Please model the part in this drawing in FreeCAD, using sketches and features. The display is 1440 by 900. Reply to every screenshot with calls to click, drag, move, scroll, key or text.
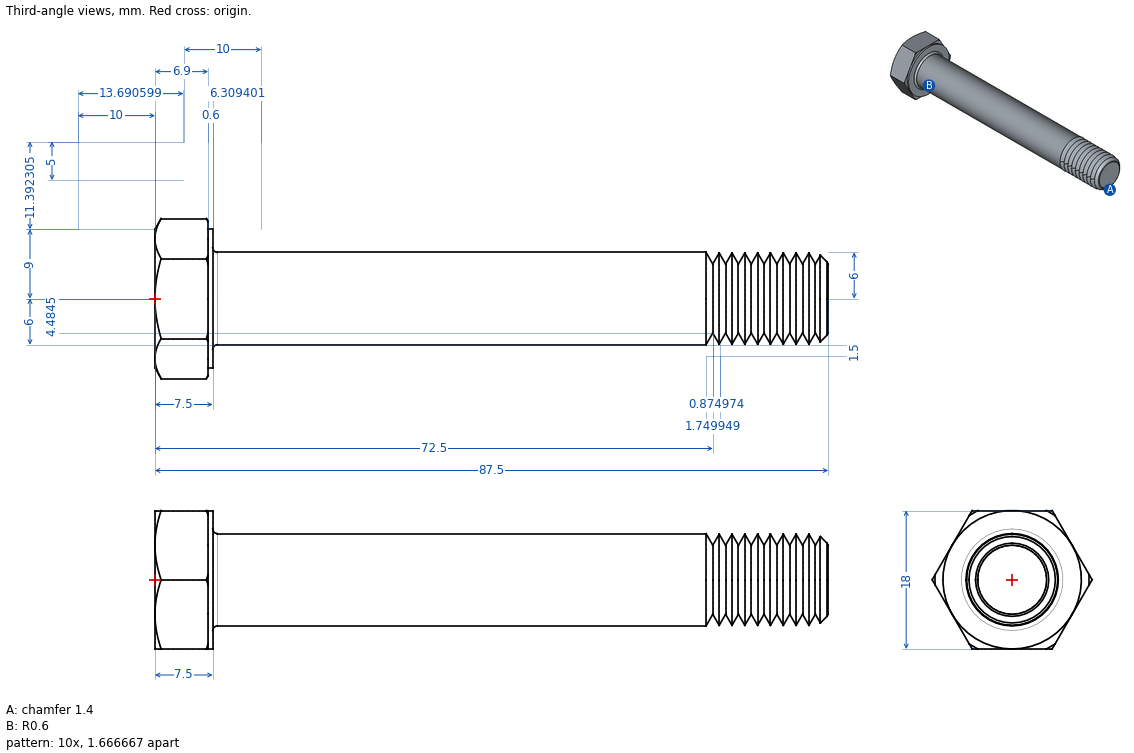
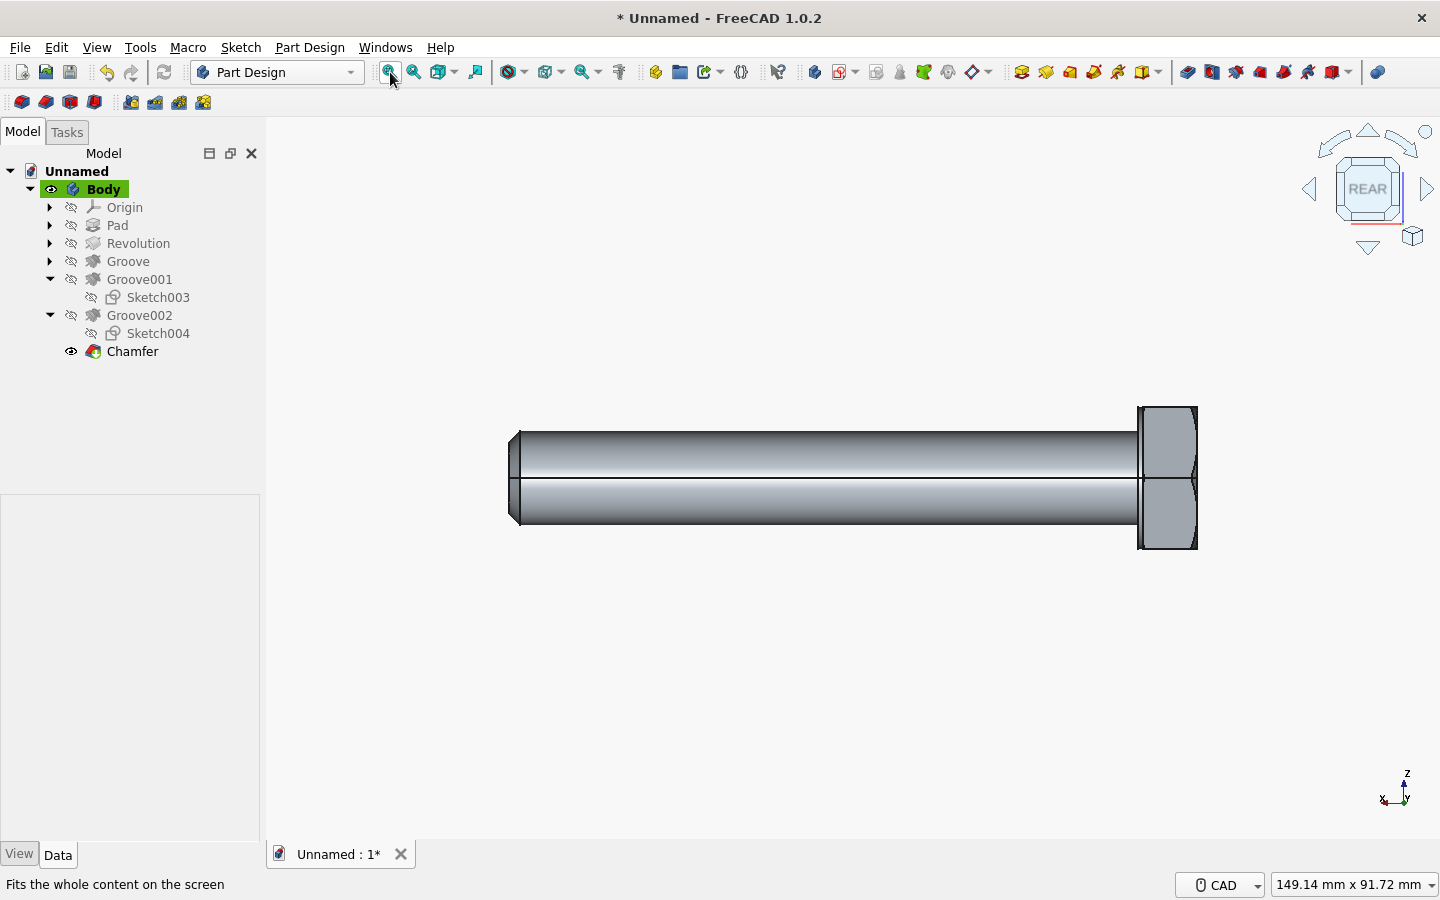
key(6)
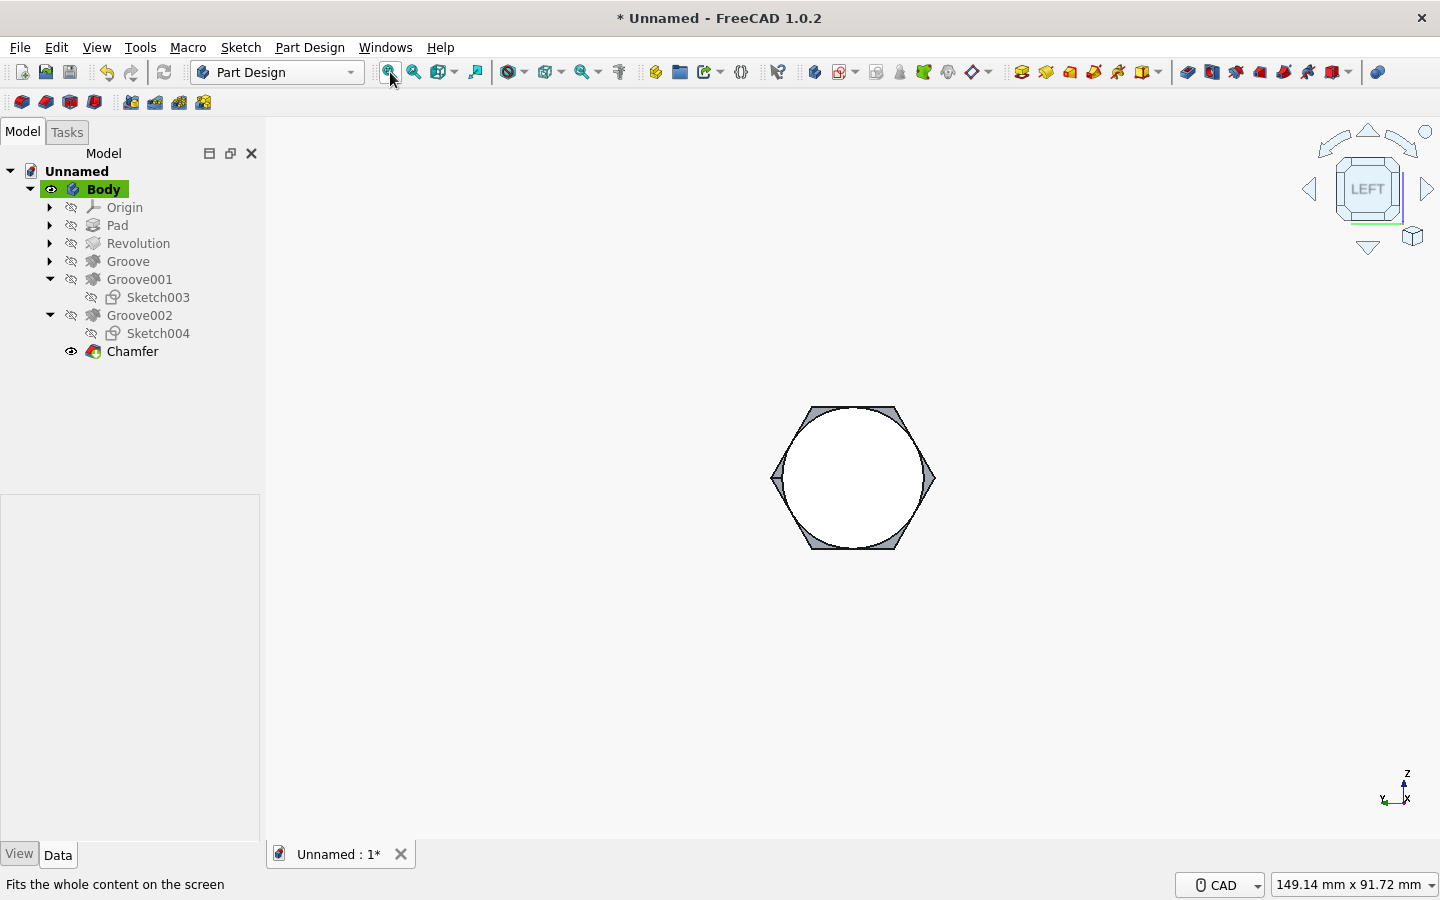
click(390, 72)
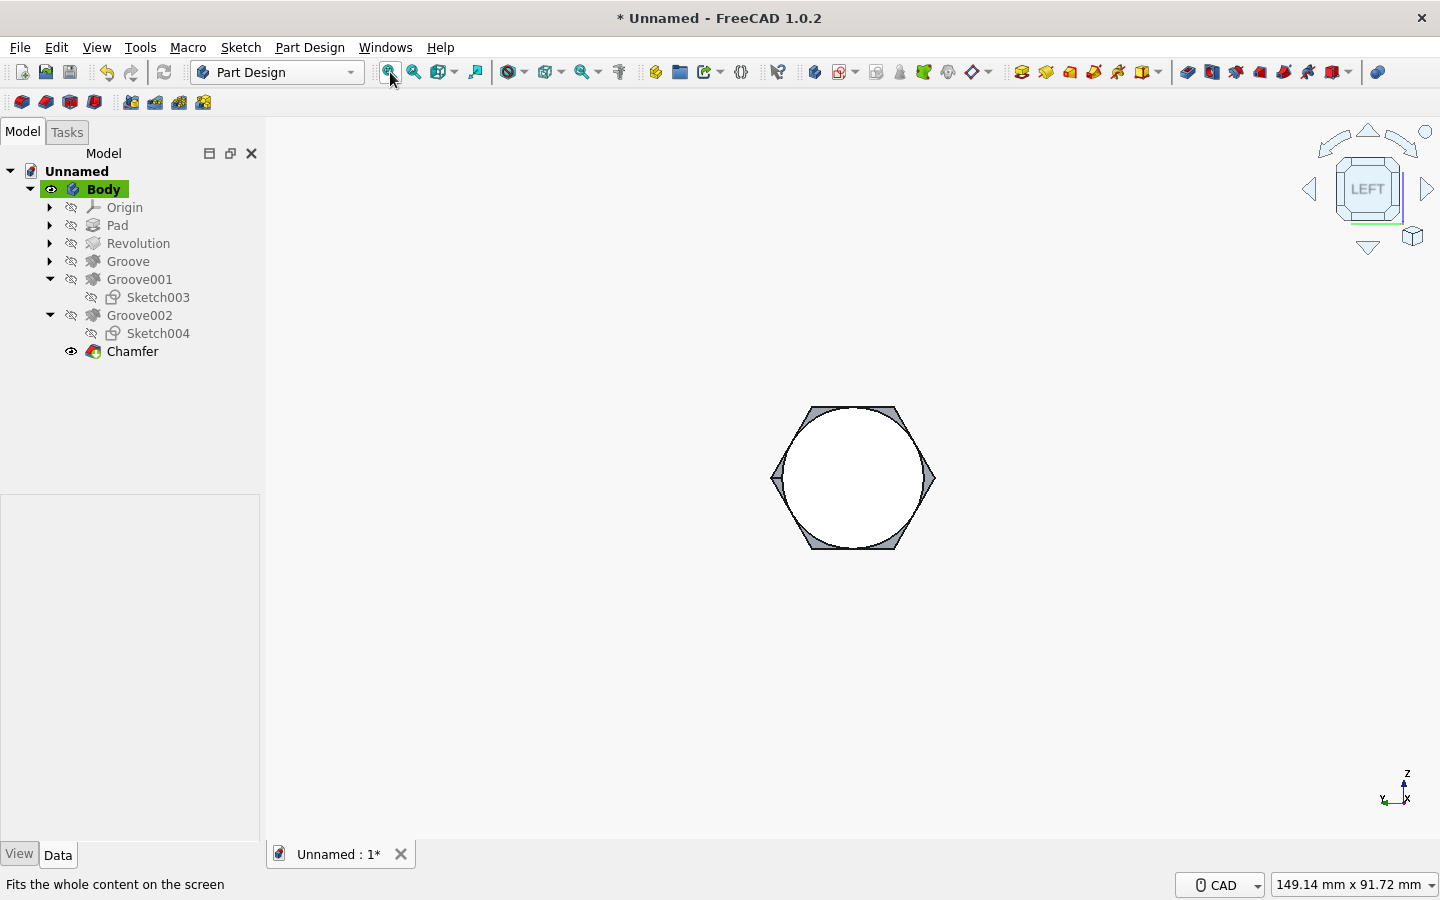
key(v)
key(3)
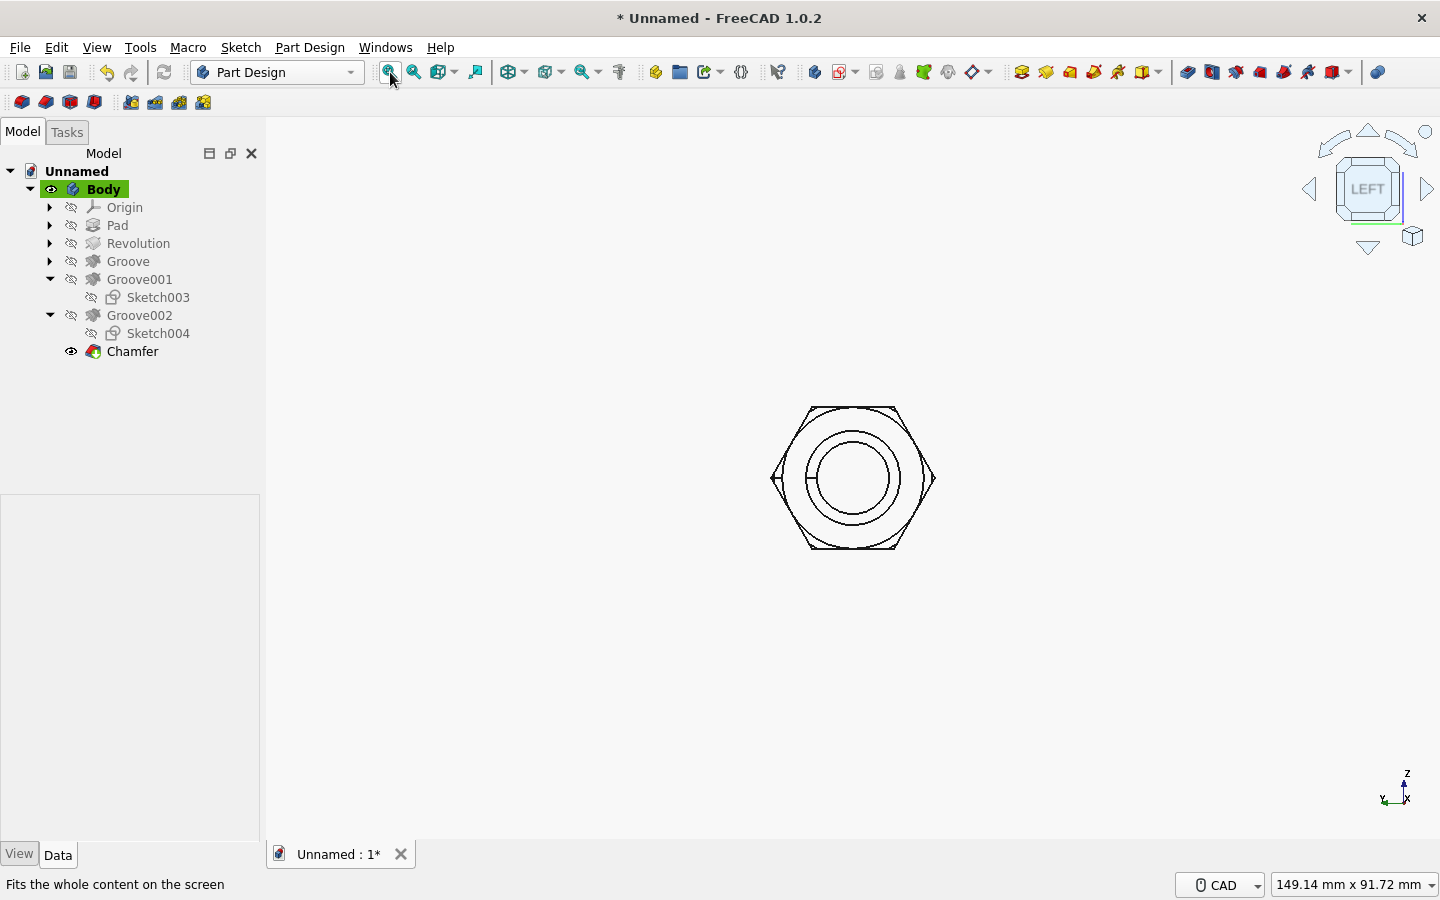
key(0)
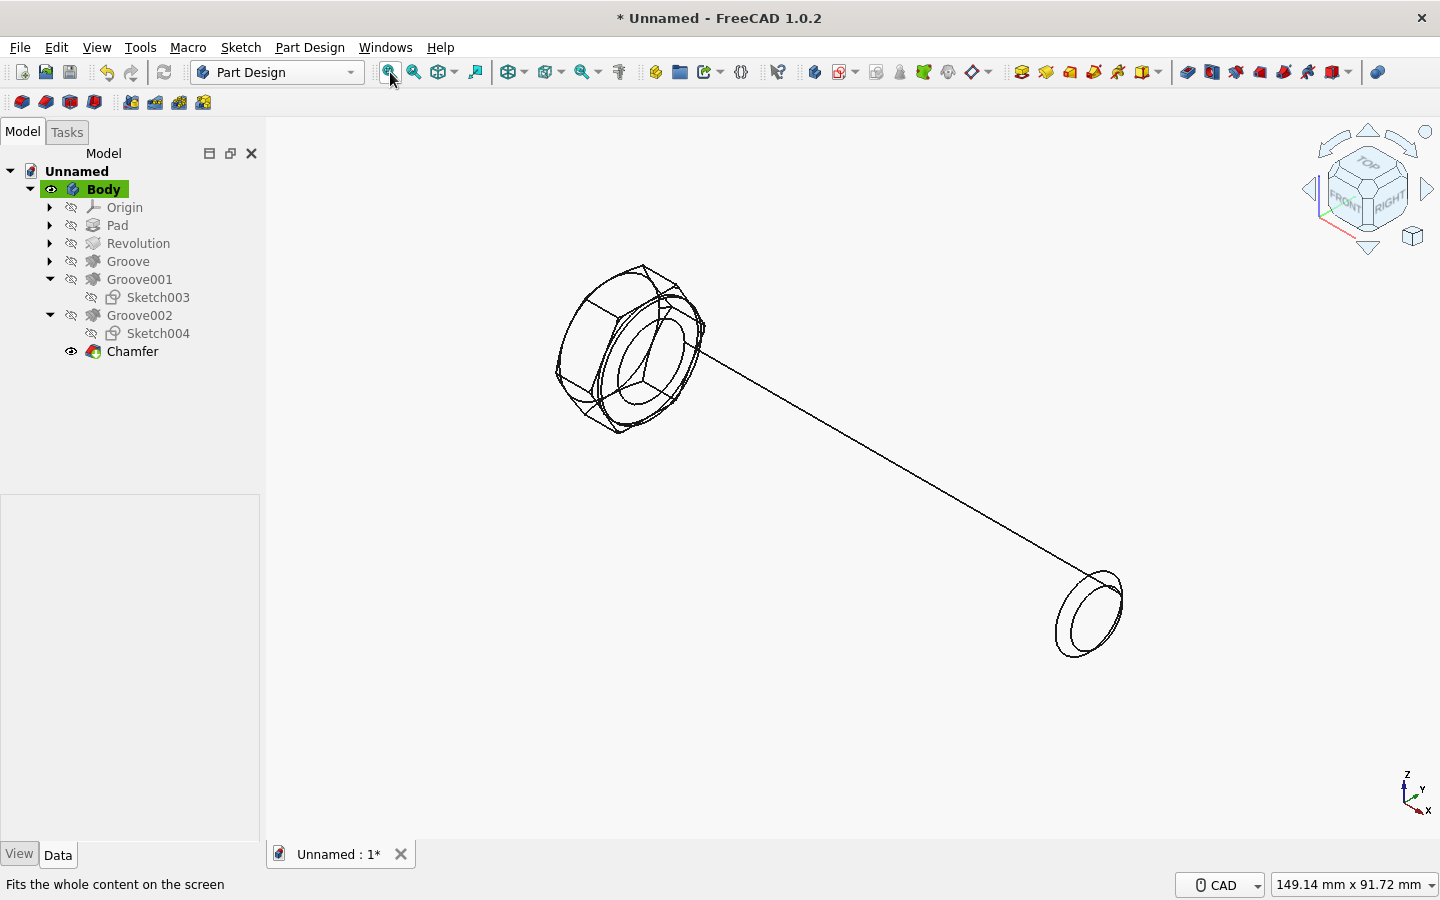
click(618, 380)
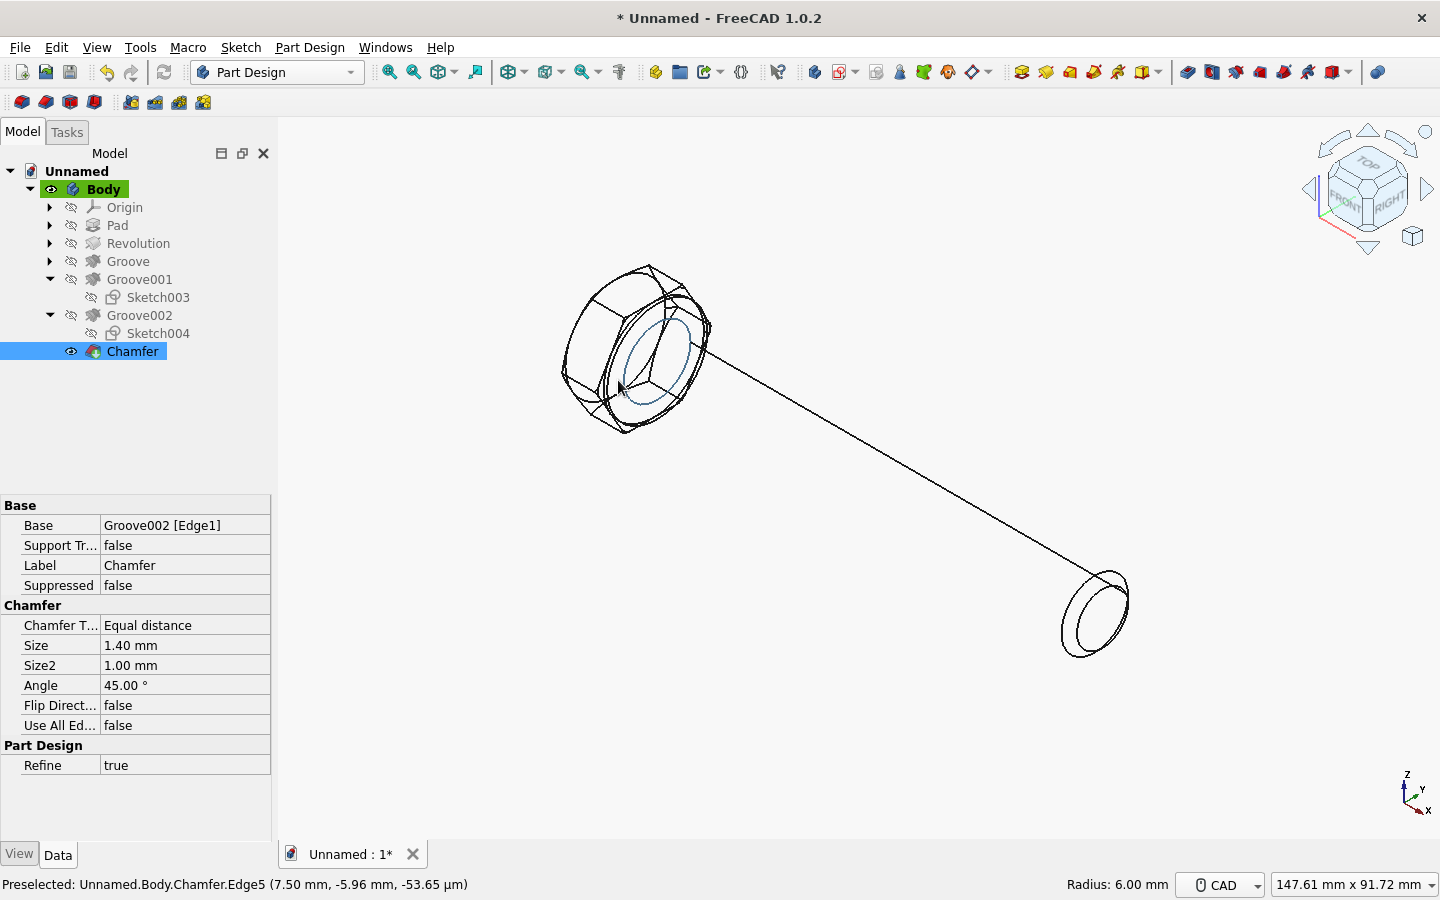
key(v)
key(1)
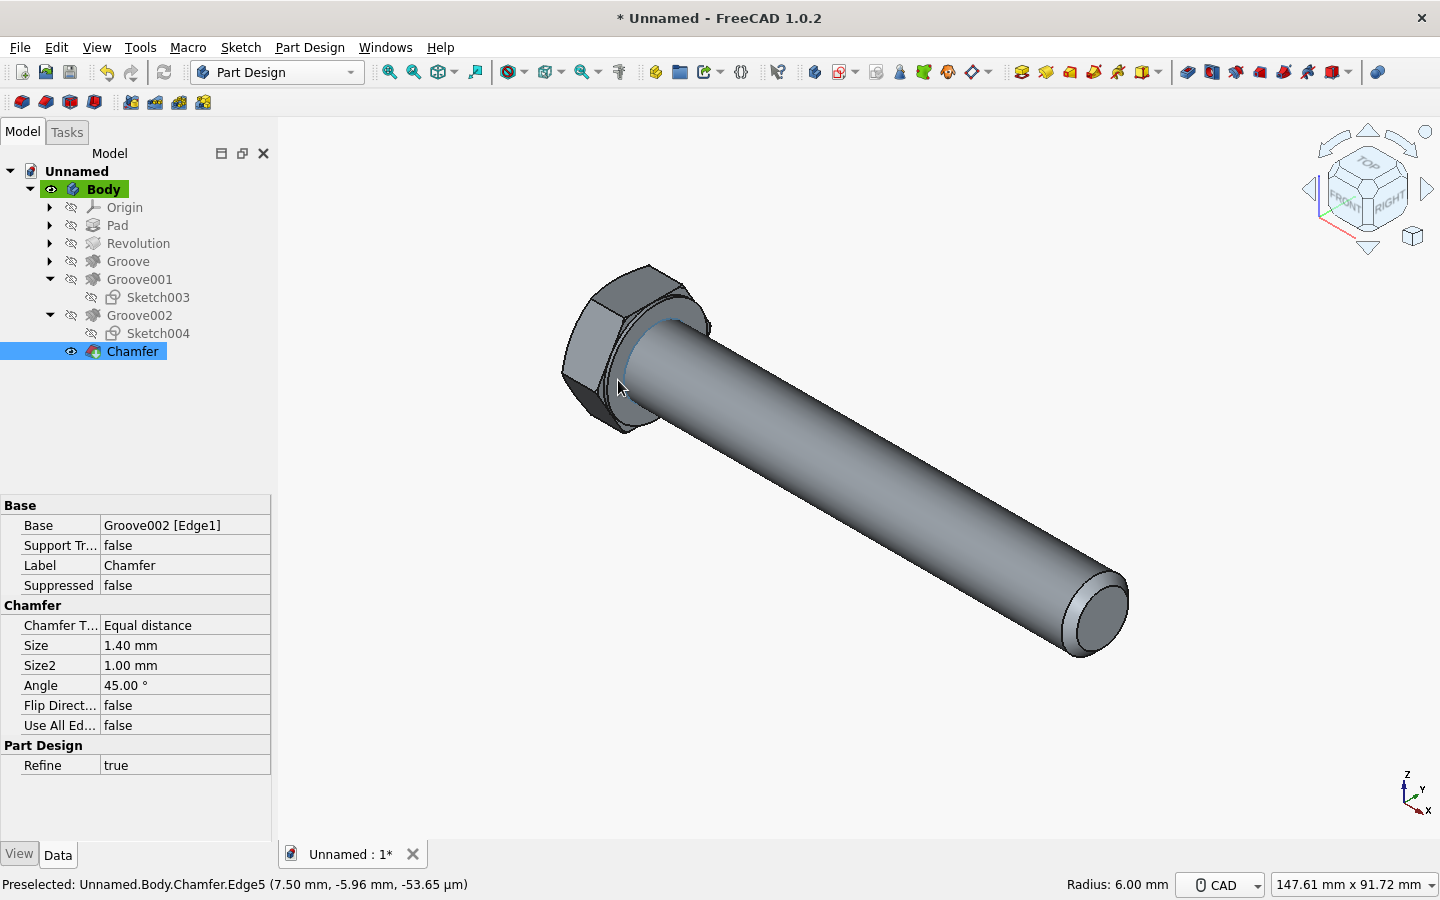
click(22, 102)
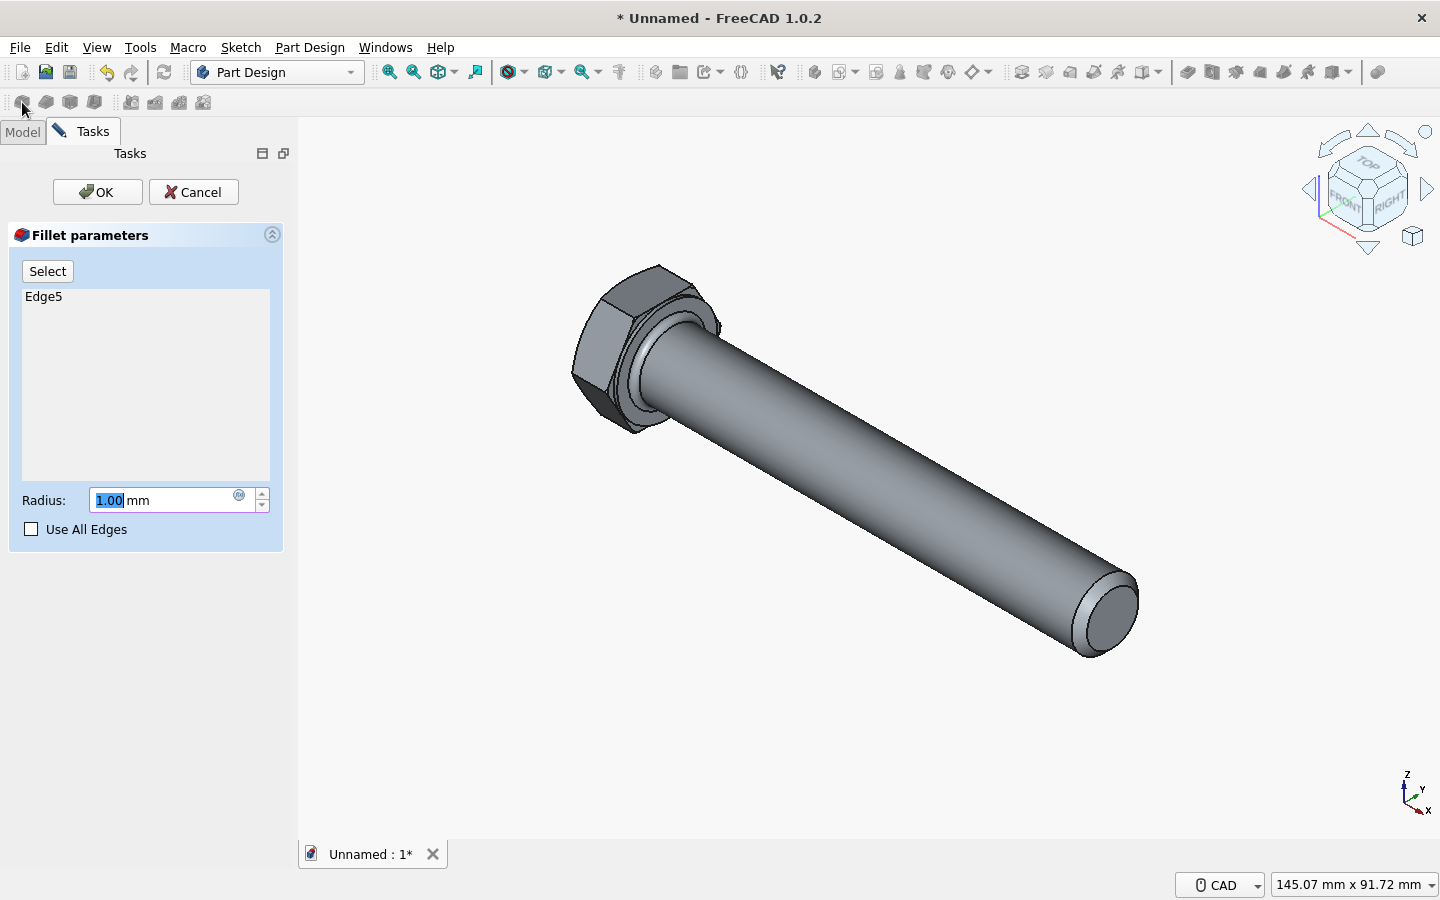
text(0.6)
key(Tab)